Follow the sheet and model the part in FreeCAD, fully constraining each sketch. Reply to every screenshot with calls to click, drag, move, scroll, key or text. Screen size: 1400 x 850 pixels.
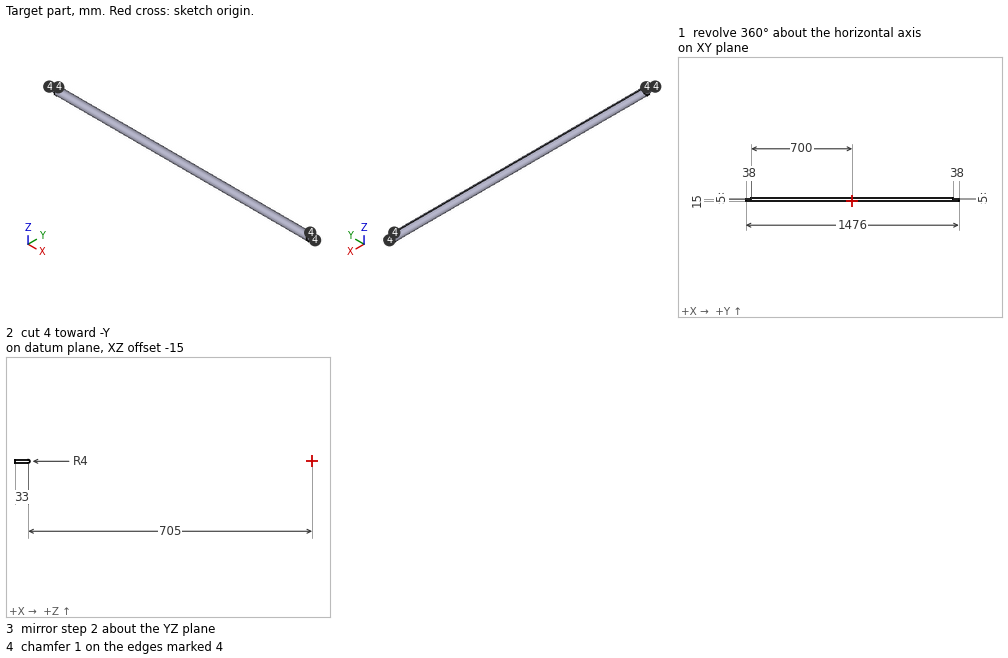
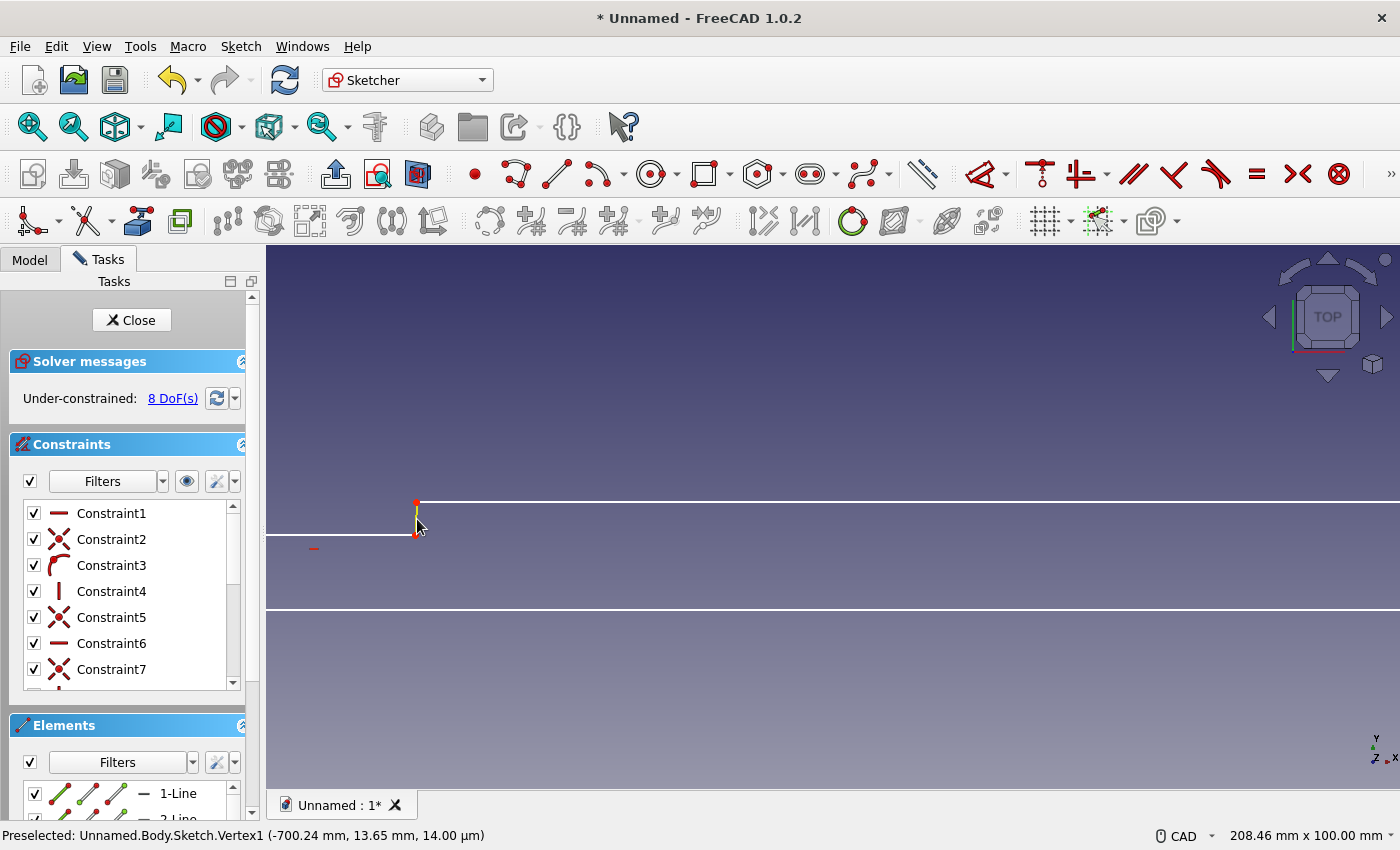
click(416, 519)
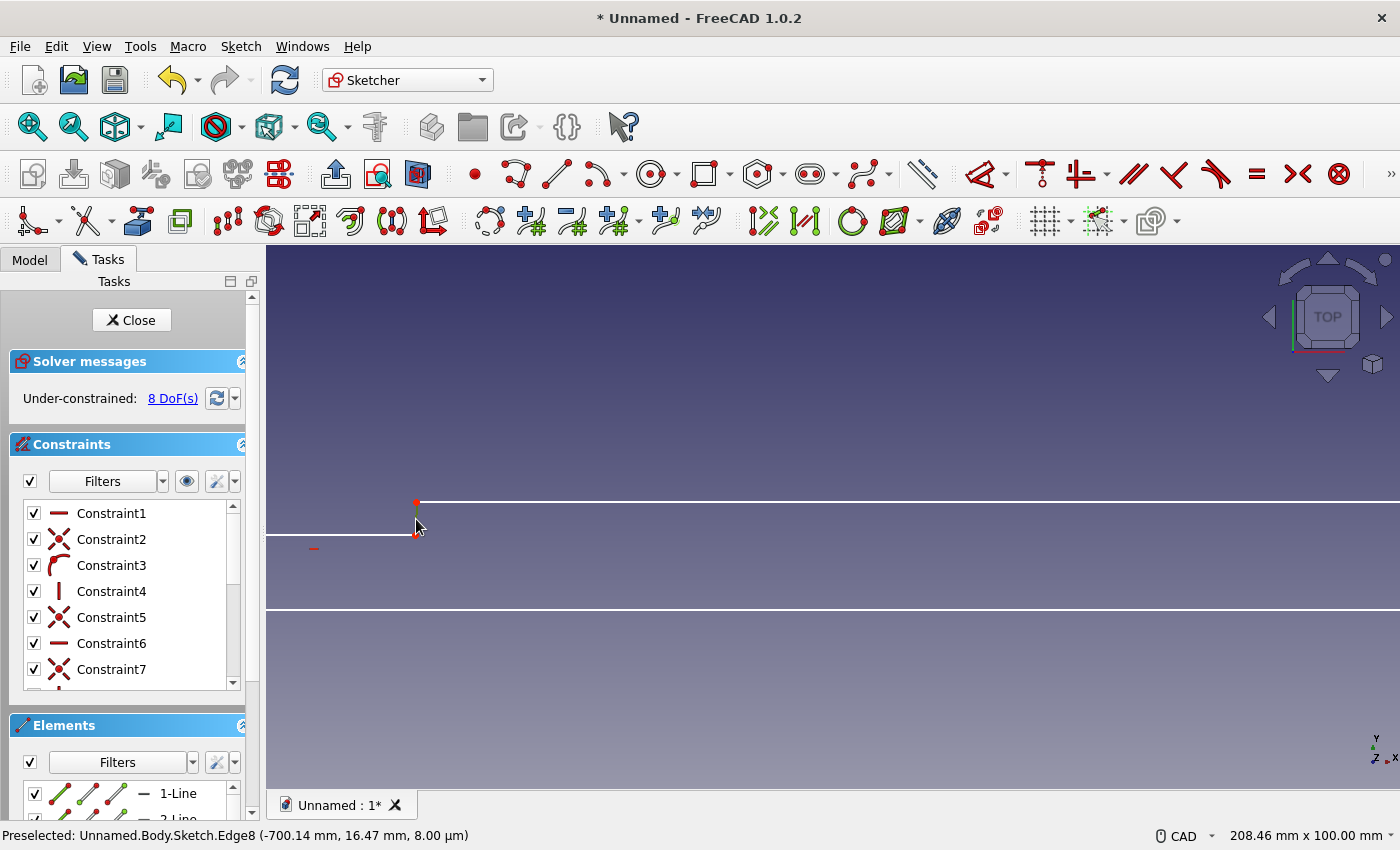
click(1106, 174)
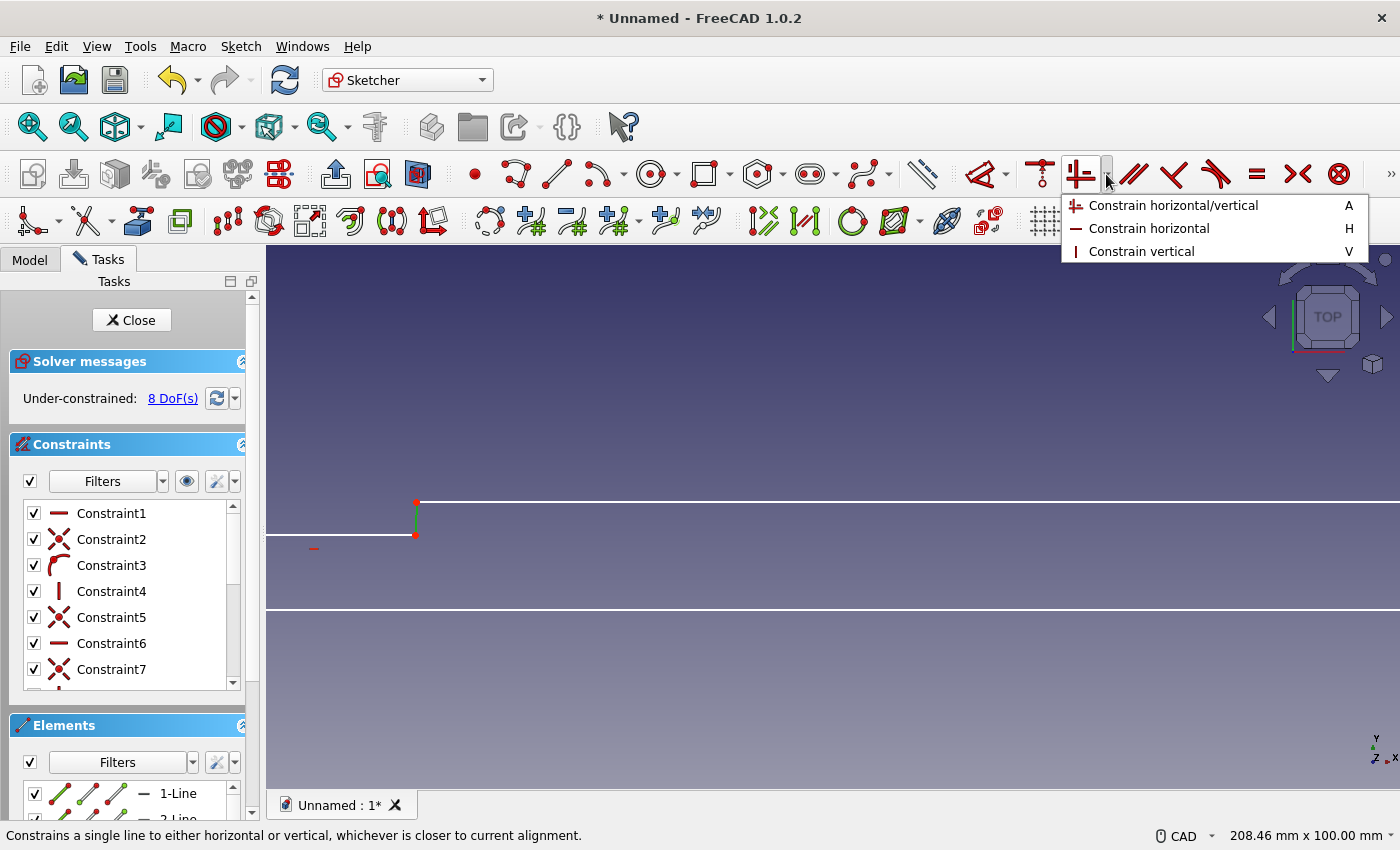
click(1215, 252)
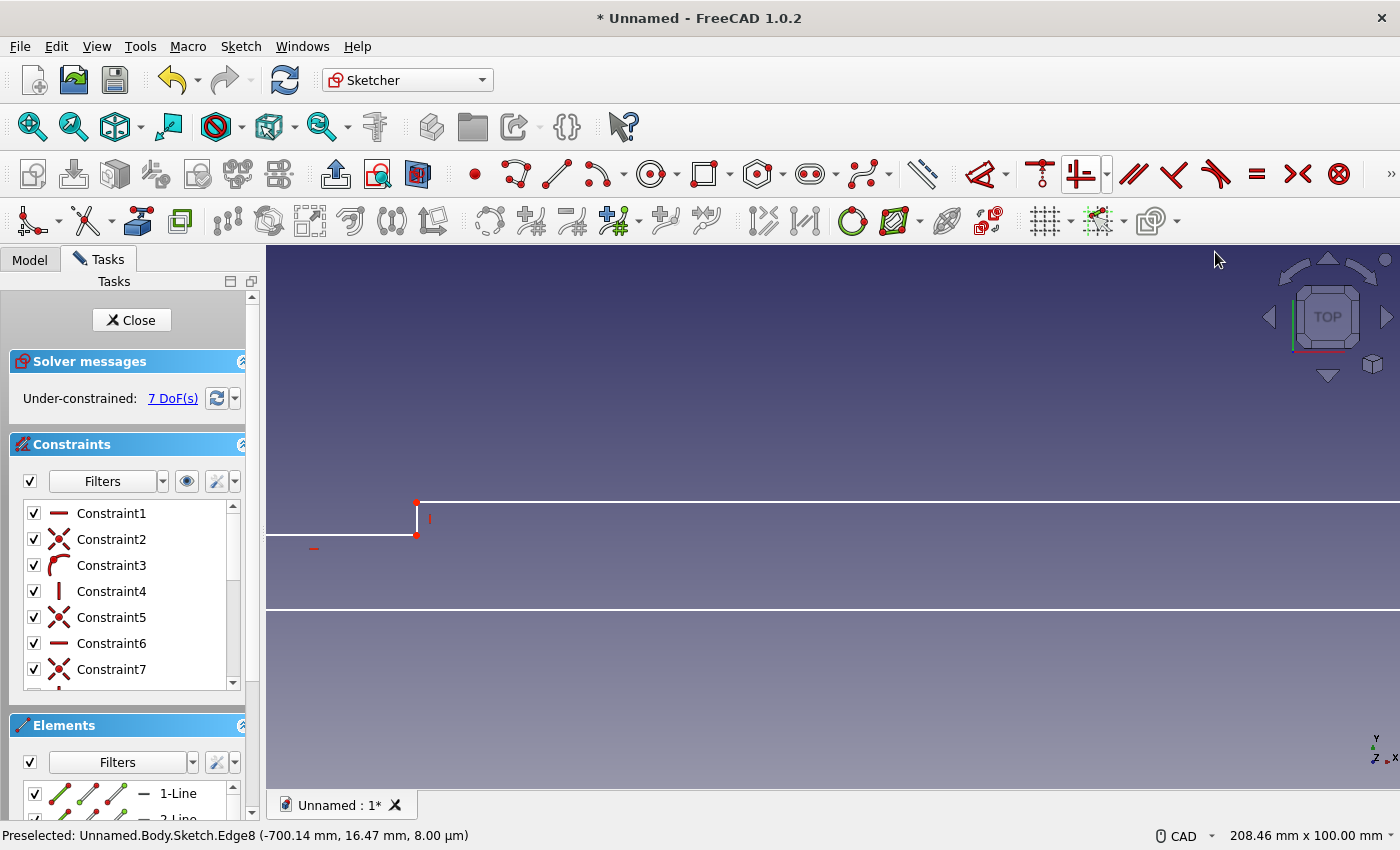
click(980, 174)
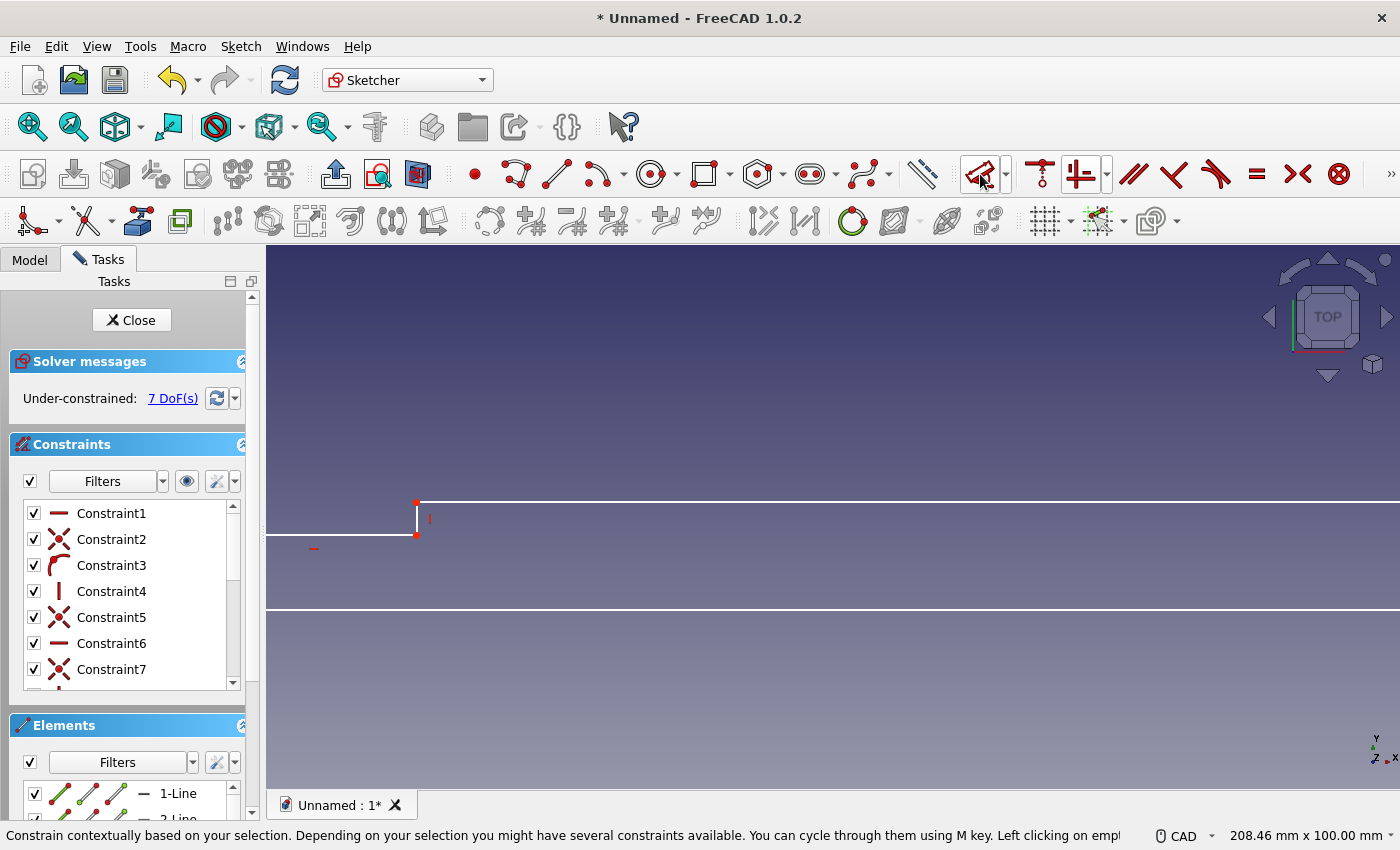
scroll(419, 513, down, 12)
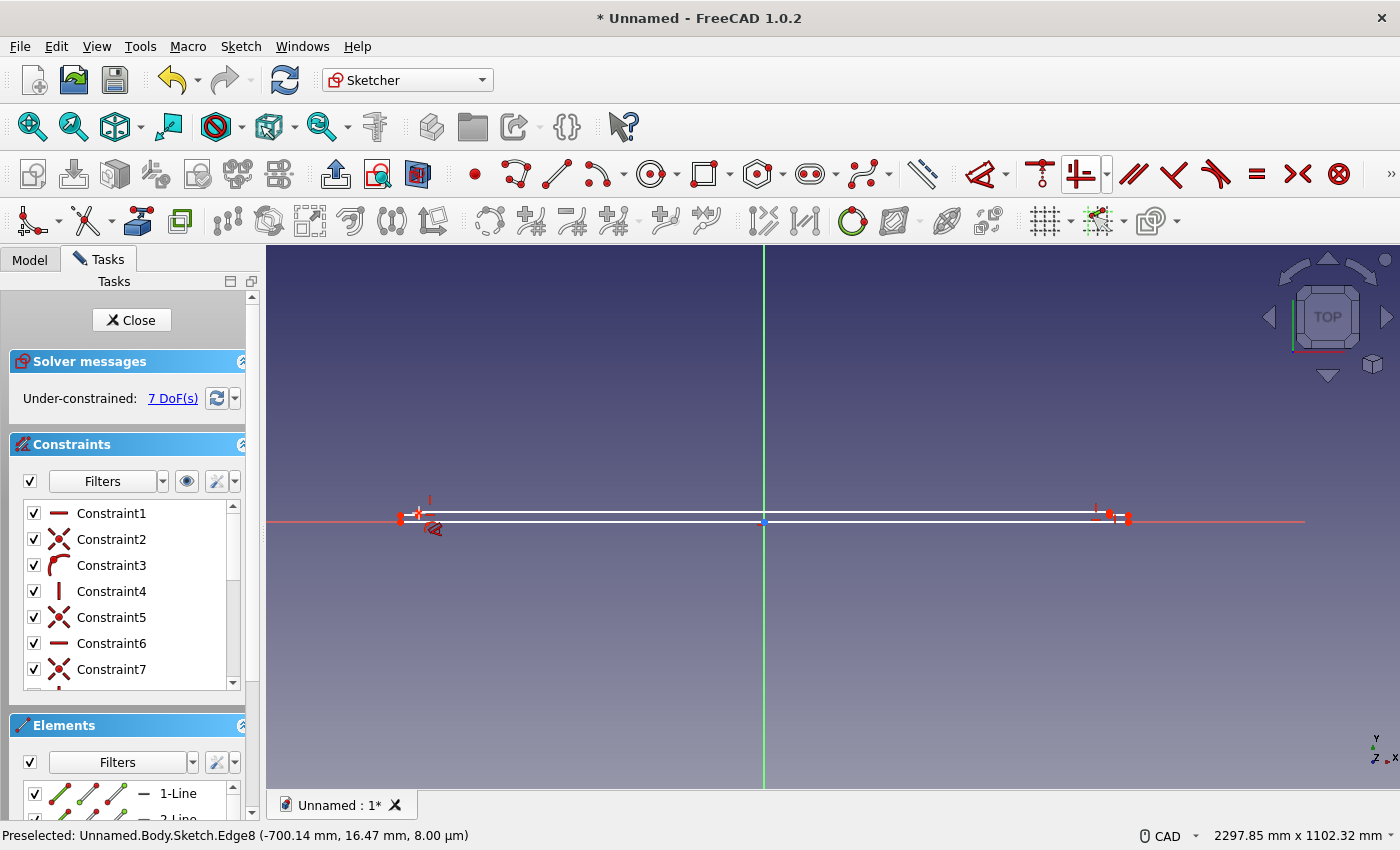
scroll(1110, 515, up, 14)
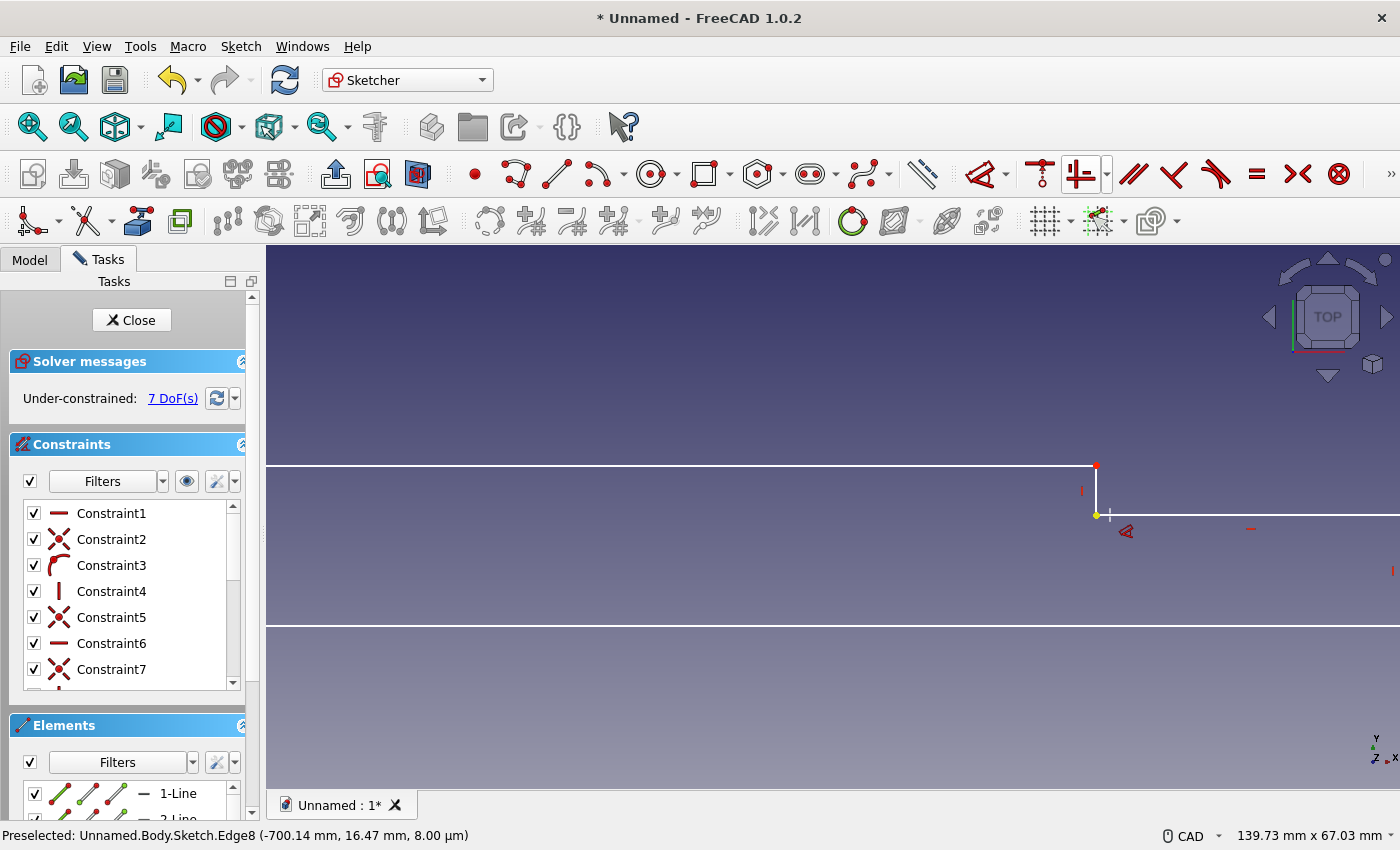
click(1096, 500)
click(1130, 491)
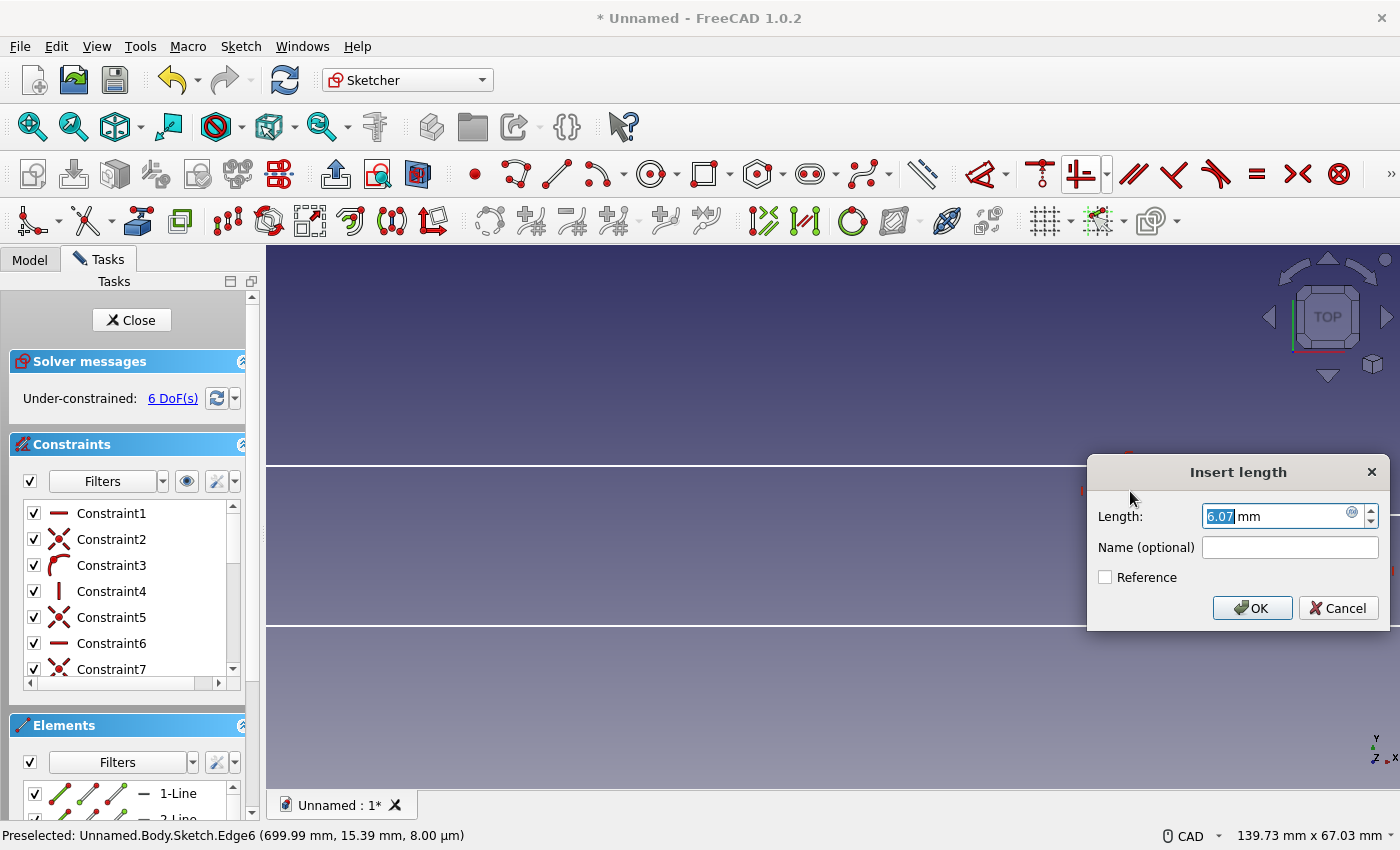
text(5)
key(Return)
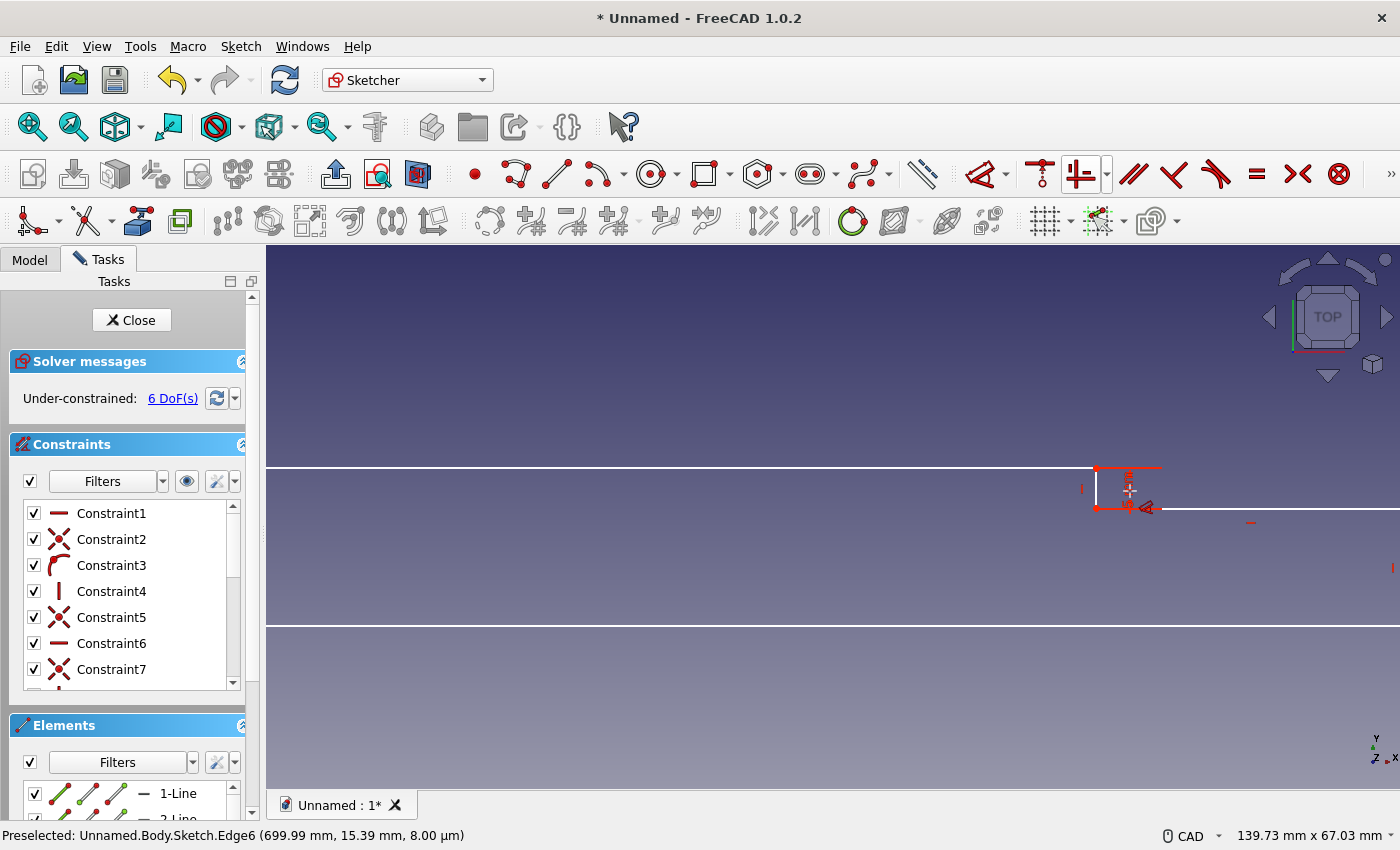
scroll(1111, 515, down, 14)